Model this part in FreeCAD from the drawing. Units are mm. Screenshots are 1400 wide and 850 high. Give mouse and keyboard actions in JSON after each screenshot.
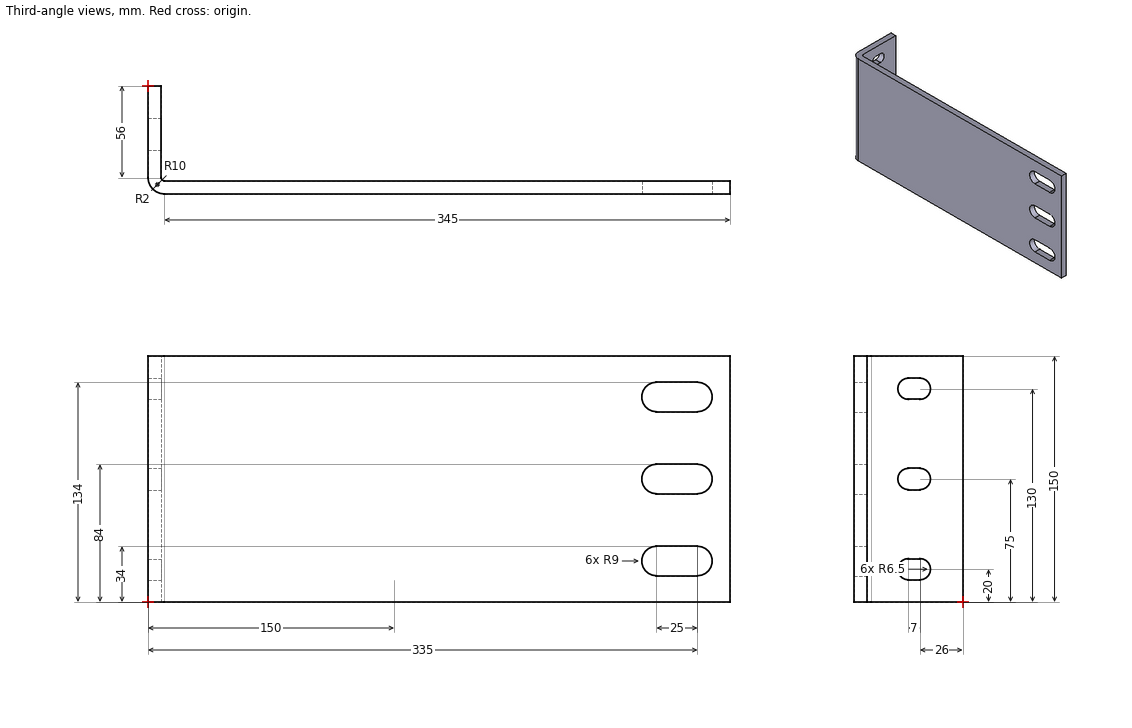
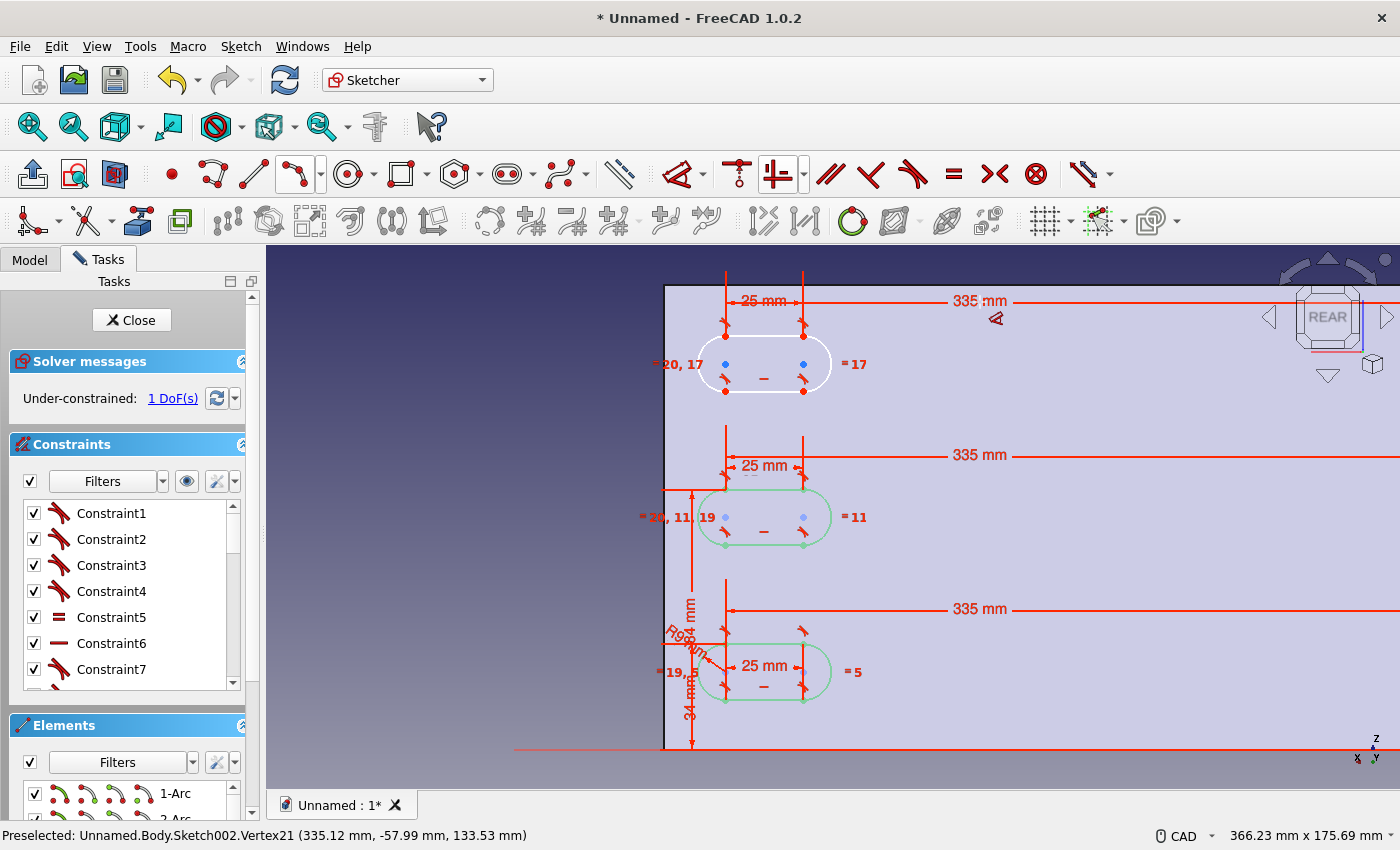
{"action": "left_click", "coordinate": [726, 336]}
{"action": "left_click", "coordinate": [692, 543]}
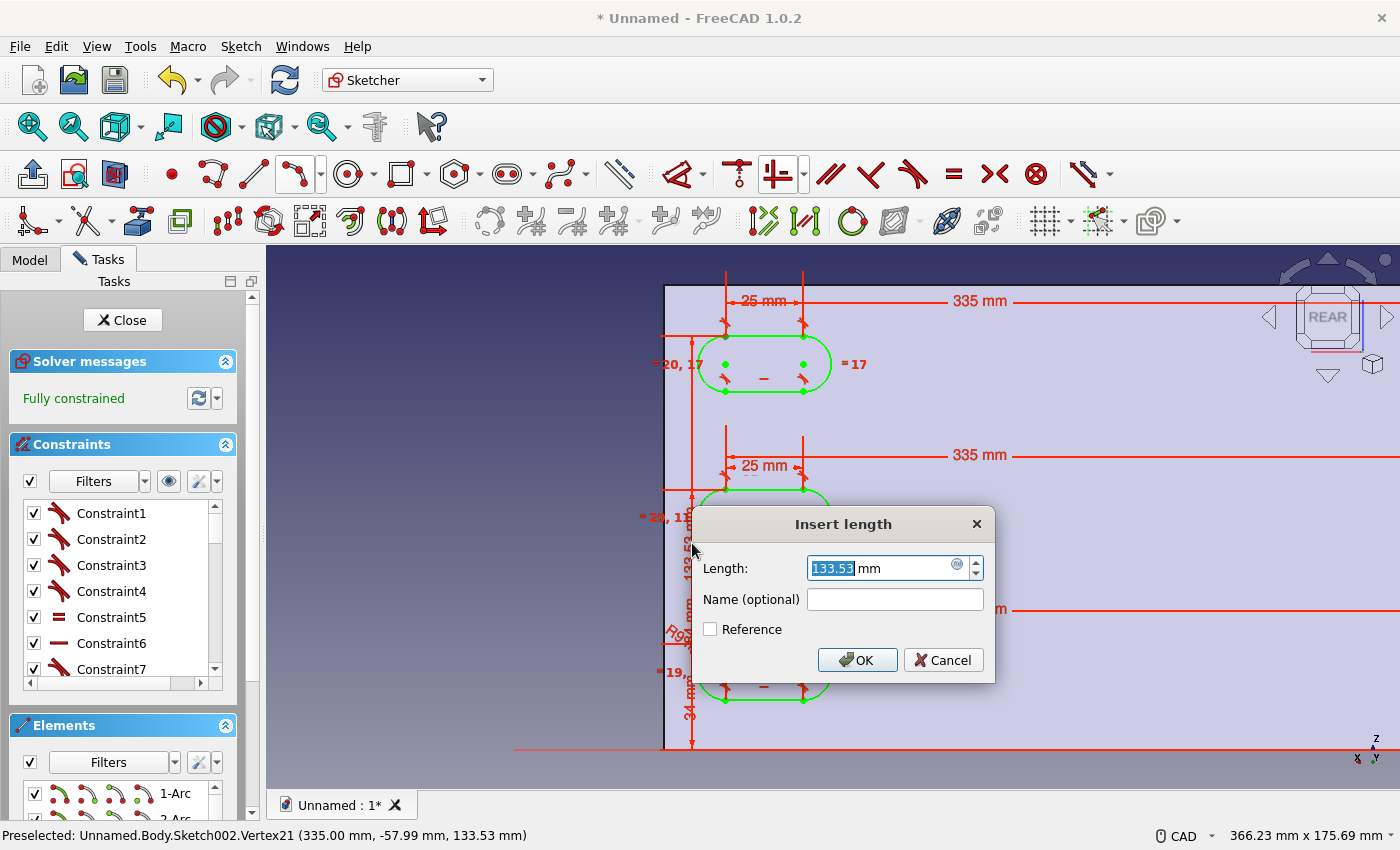
{"action": "type", "text": "134"}
{"action": "key", "text": "Return"}
{"action": "key", "text": "Escape"}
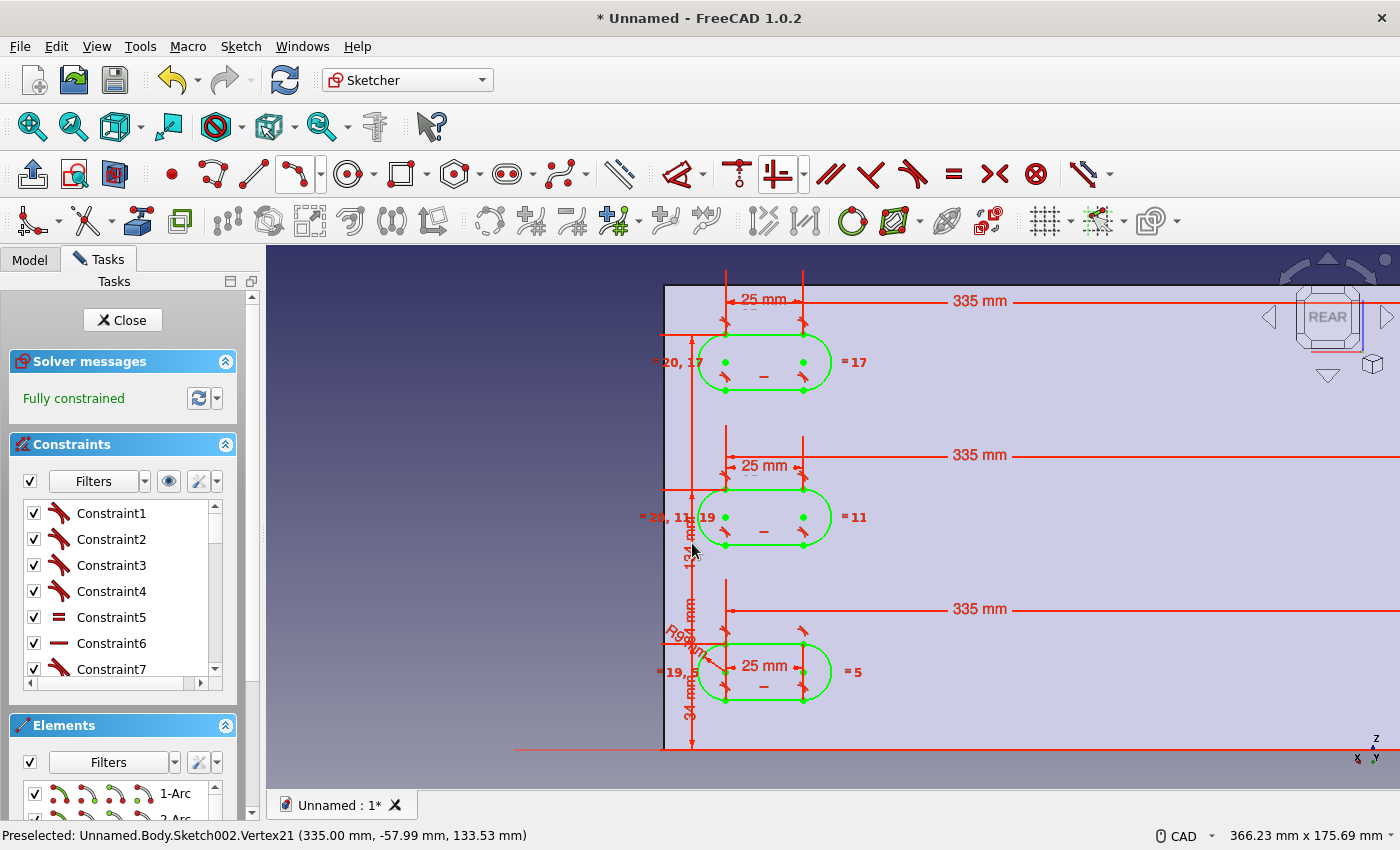
{"action": "left_click", "coordinate": [123, 320]}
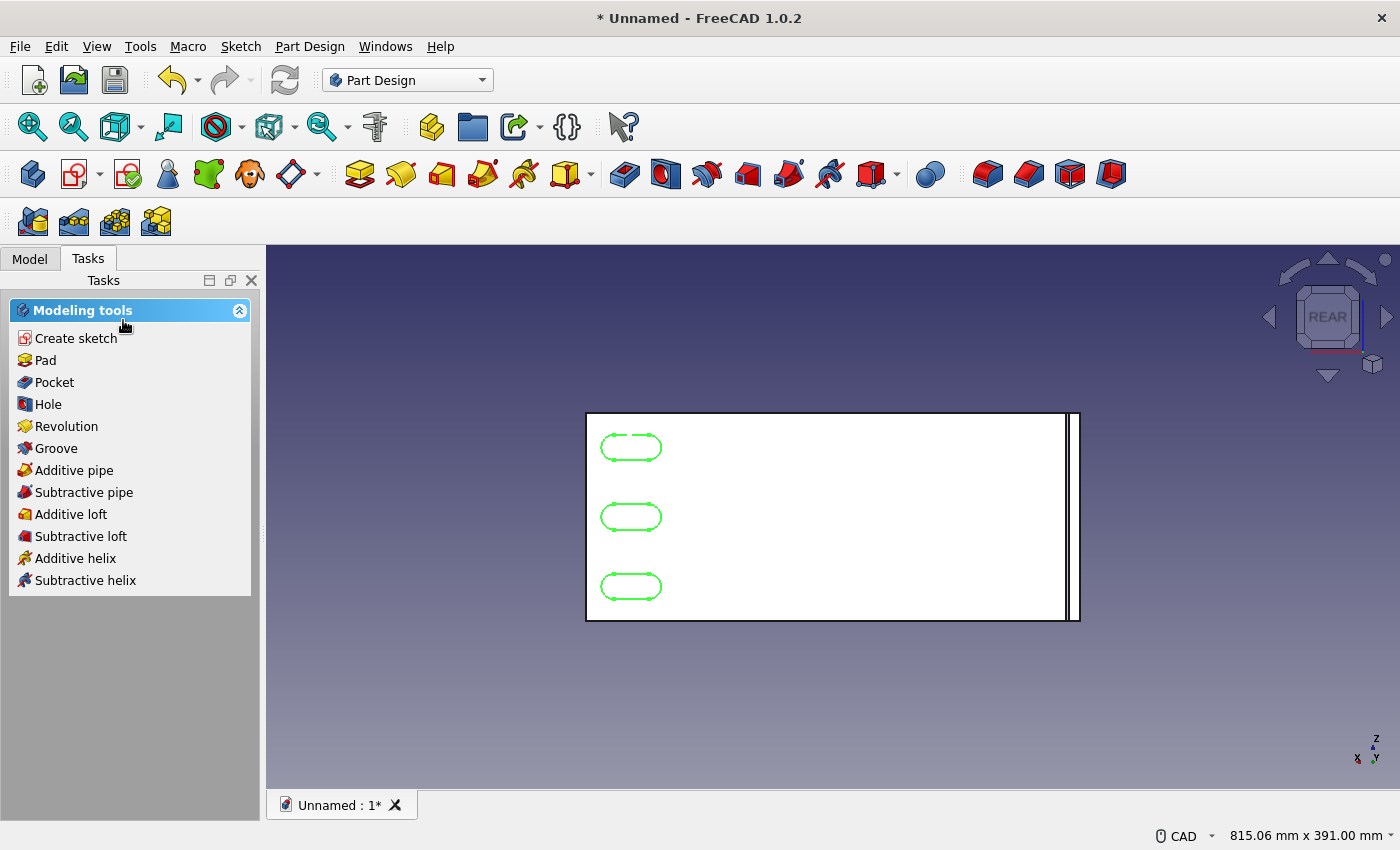
{"action": "left_click", "coordinate": [625, 174]}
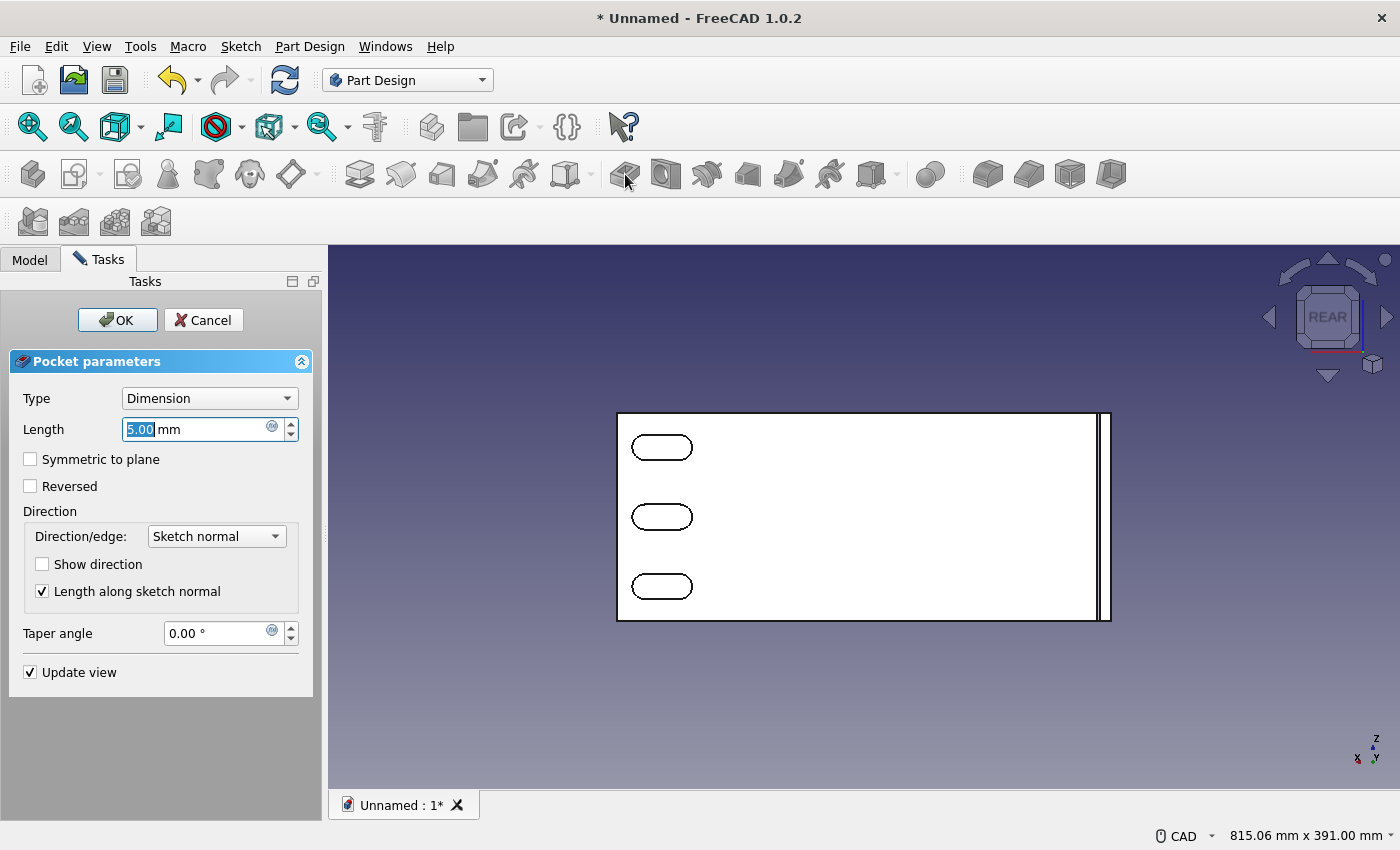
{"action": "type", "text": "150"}
{"action": "key", "text": "Tab"}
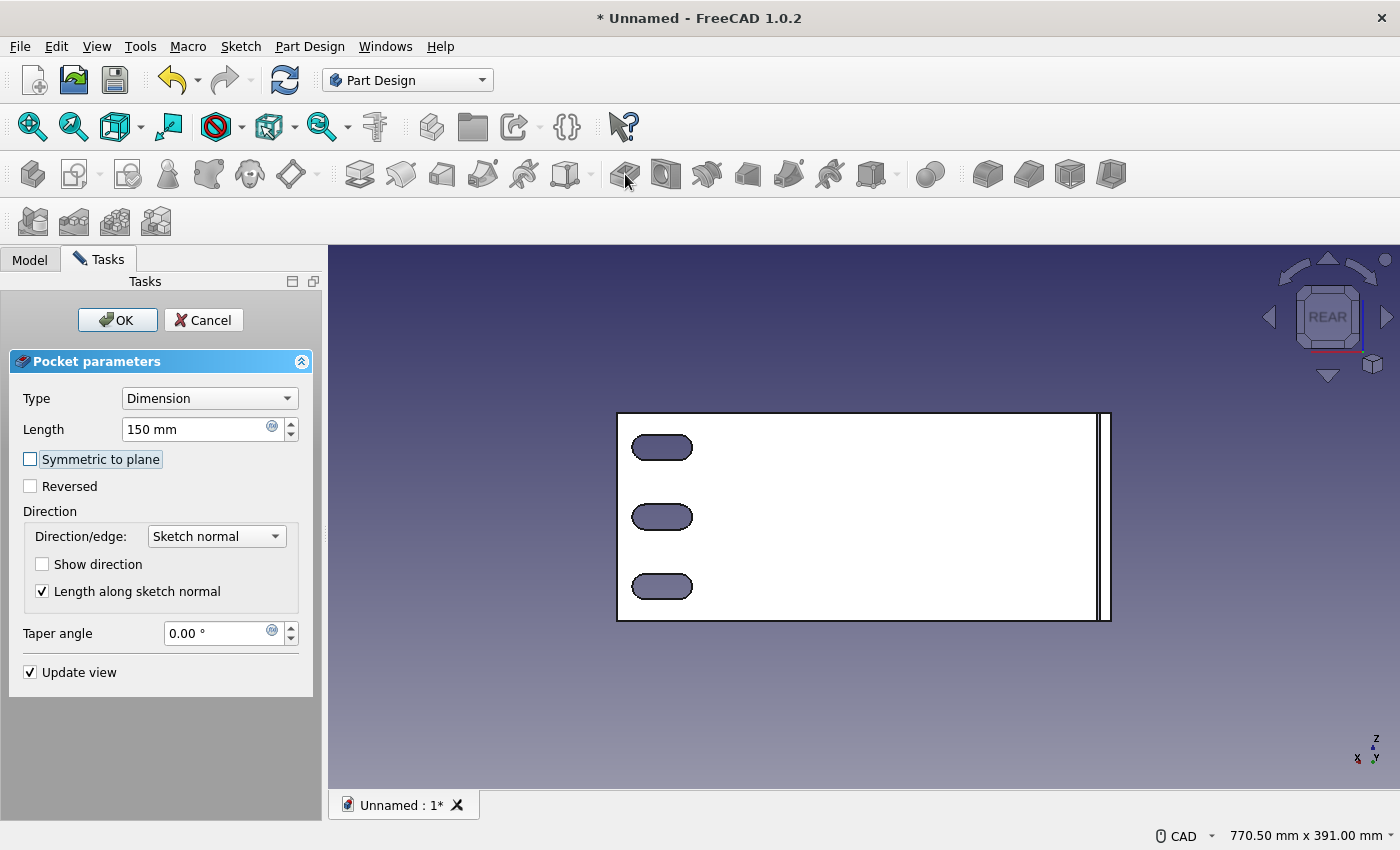
{"action": "left_click", "coordinate": [118, 320]}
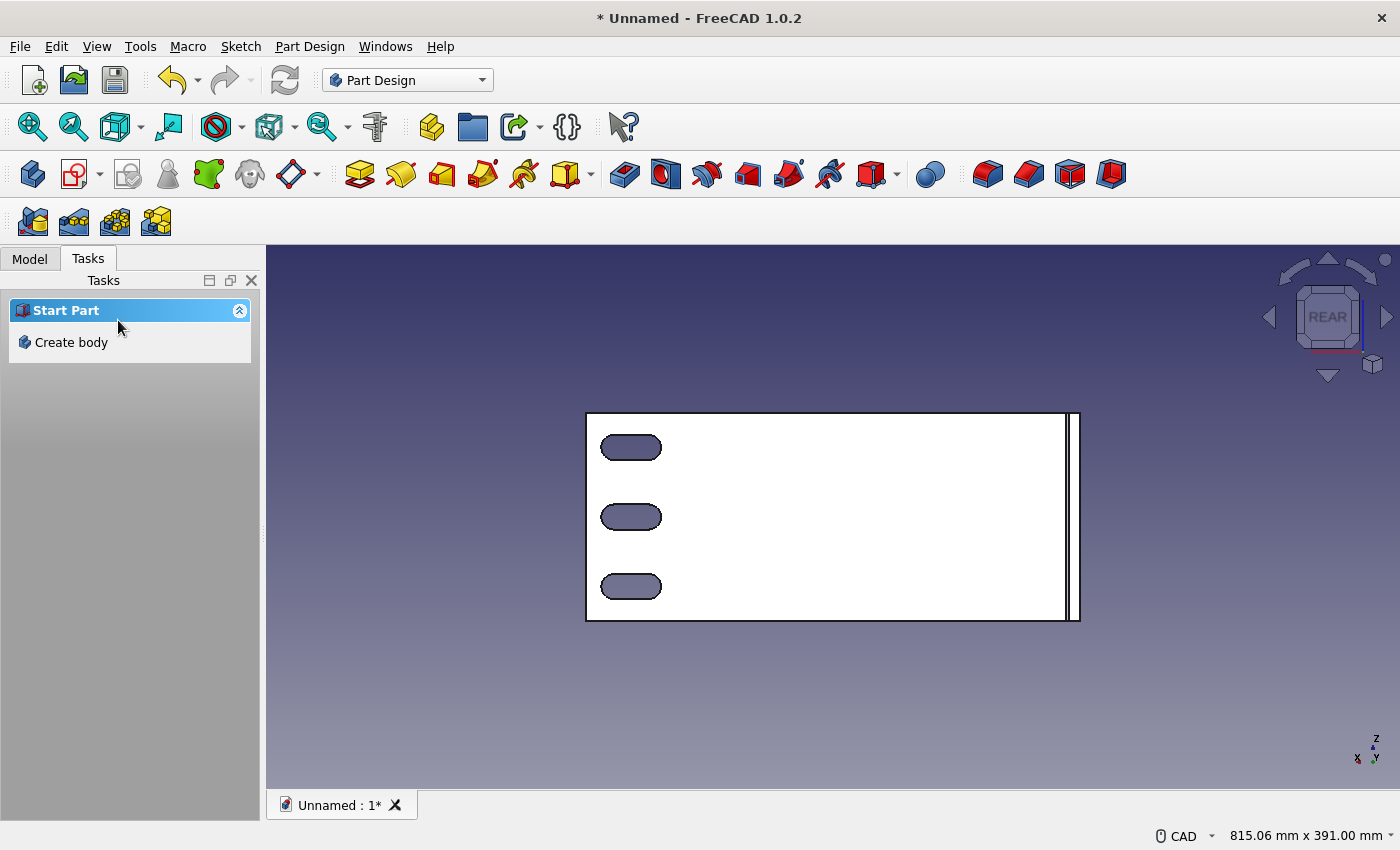
{"action": "key", "text": "0"}